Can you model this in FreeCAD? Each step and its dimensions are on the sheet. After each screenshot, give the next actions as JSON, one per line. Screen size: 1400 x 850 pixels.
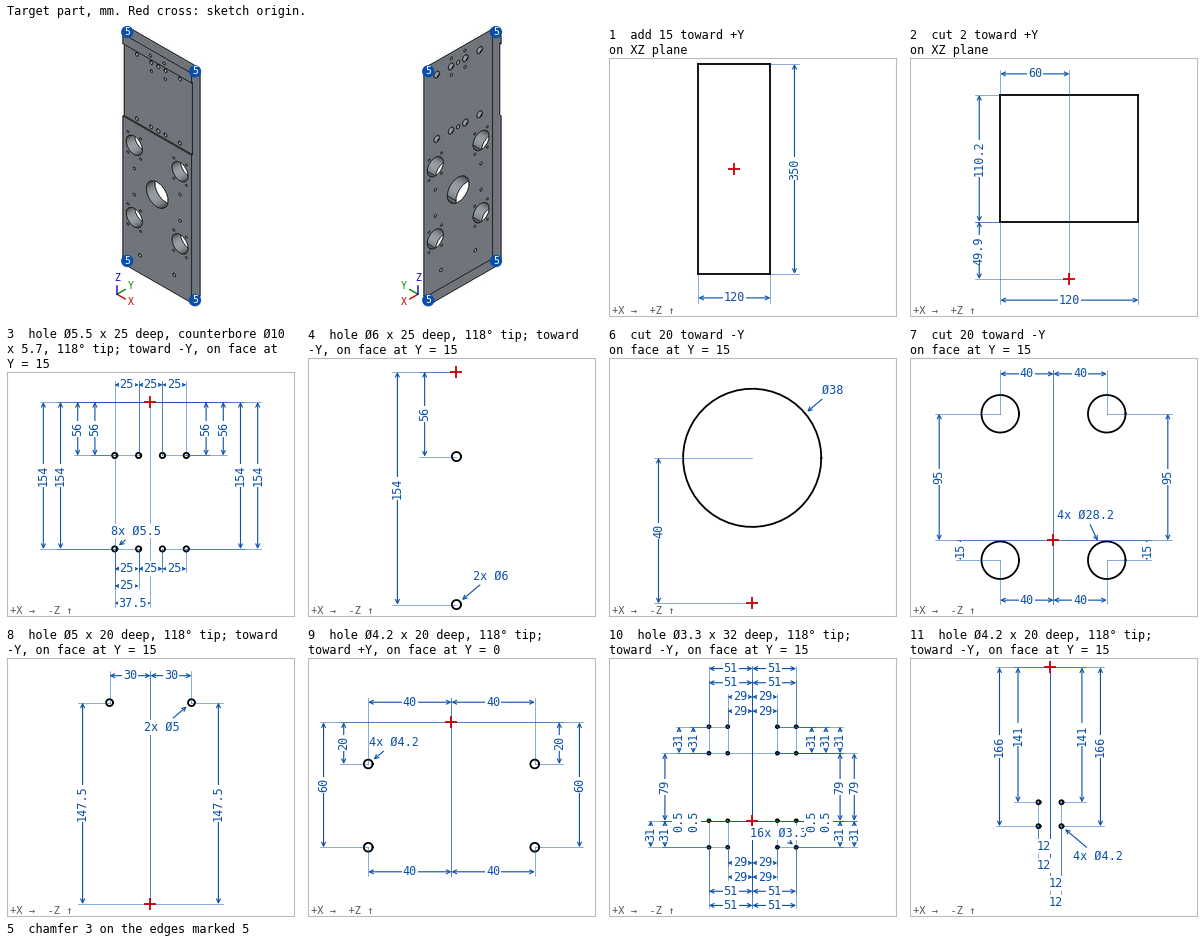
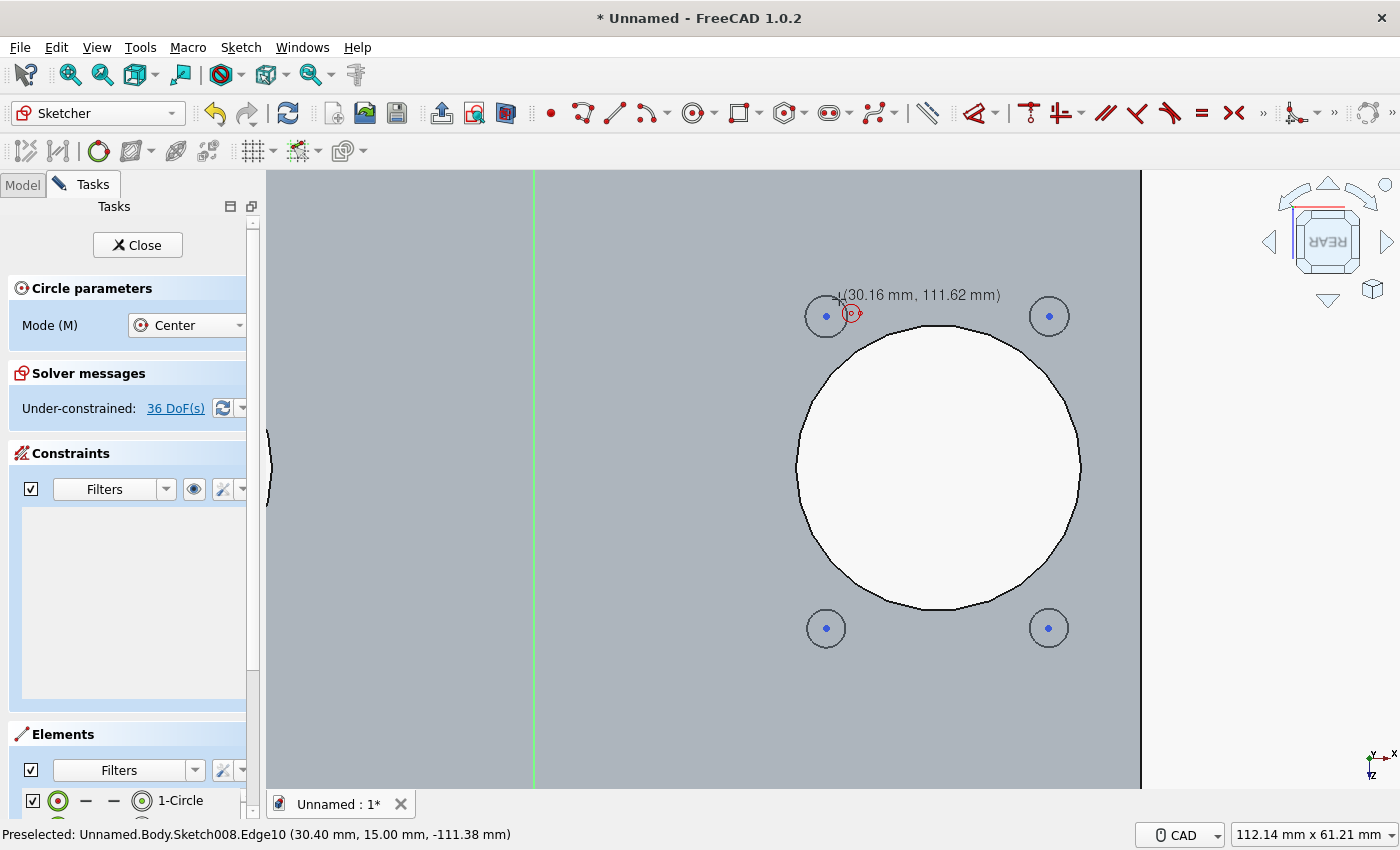
{"action": "scroll", "coordinate": [840, 301], "scroll_direction": "down", "scroll_amount": 7}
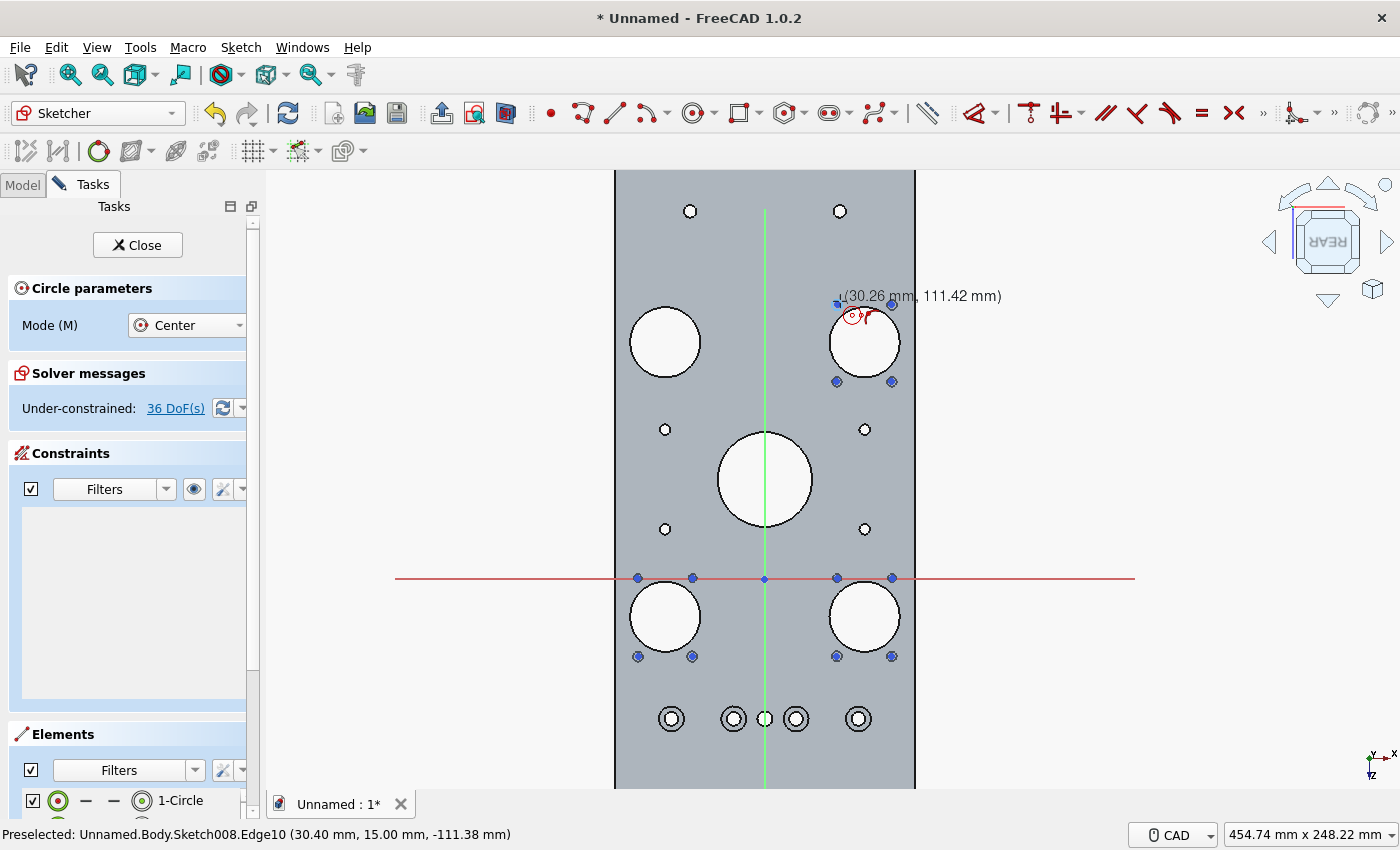
{"action": "scroll", "coordinate": [693, 381], "scroll_direction": "up", "scroll_amount": 9}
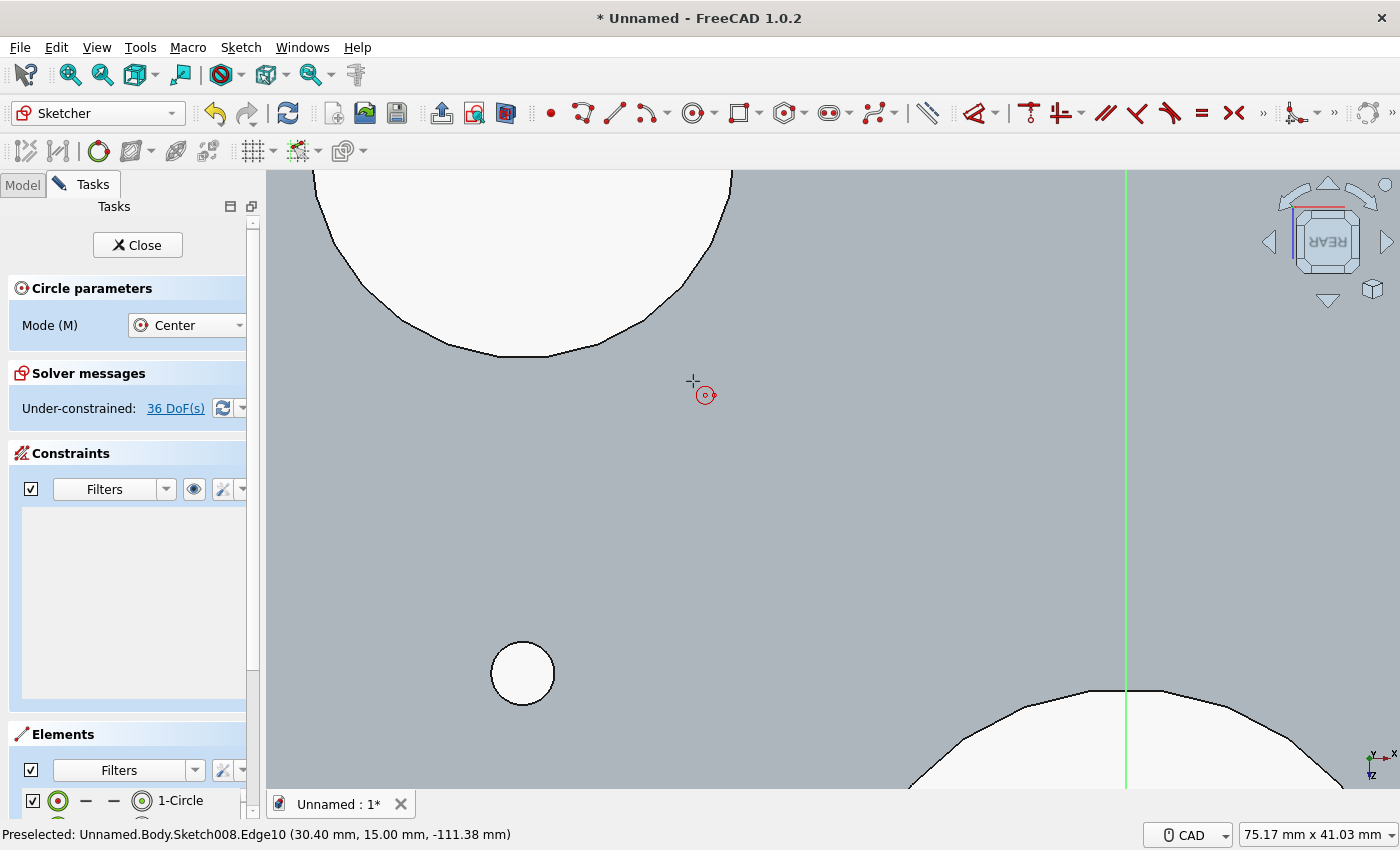
{"action": "scroll", "coordinate": [693, 381], "scroll_direction": "down", "scroll_amount": 9}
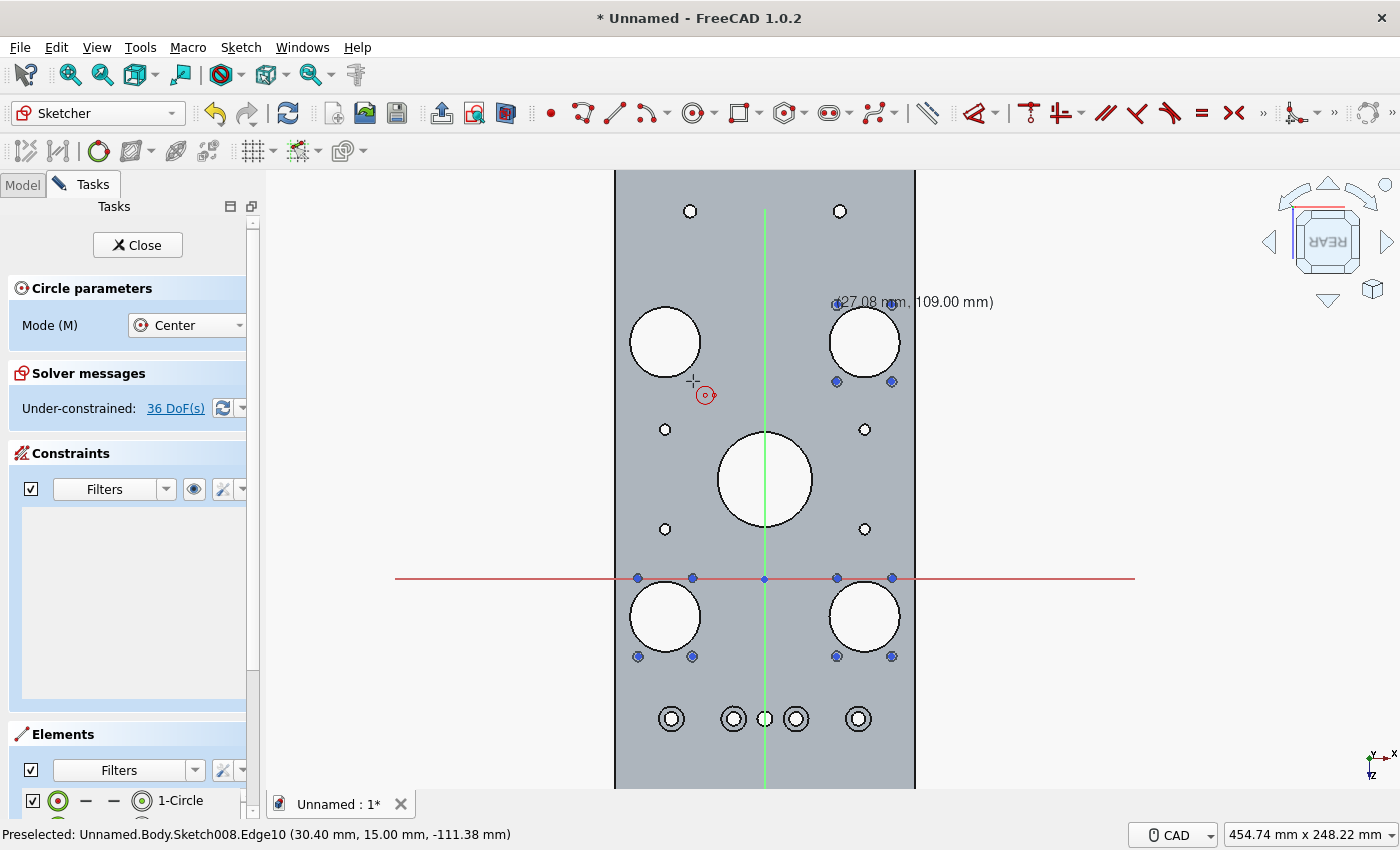
{"action": "left_click", "coordinate": [693, 381]}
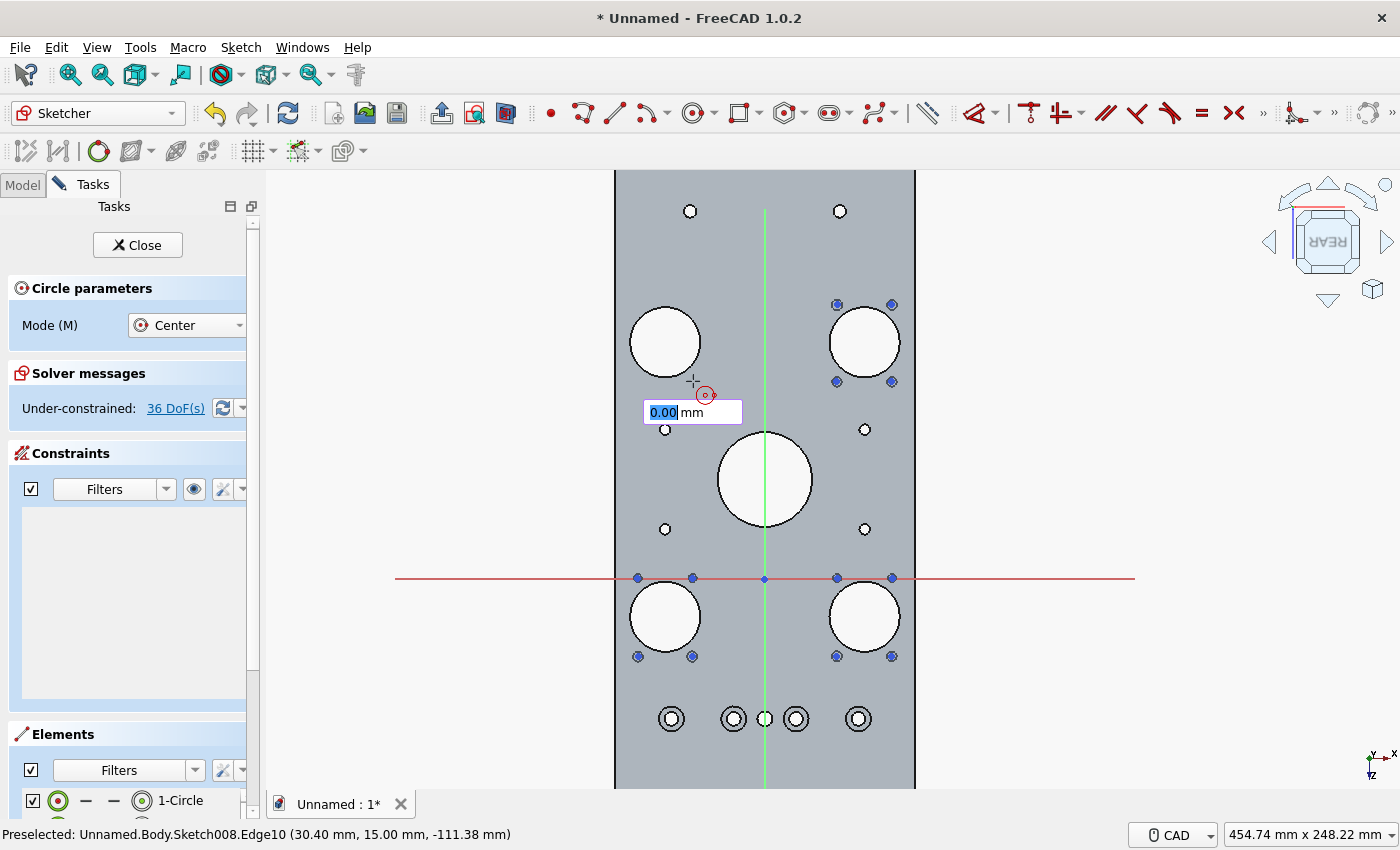
{"action": "scroll", "coordinate": [696, 378], "scroll_direction": "up", "scroll_amount": 7}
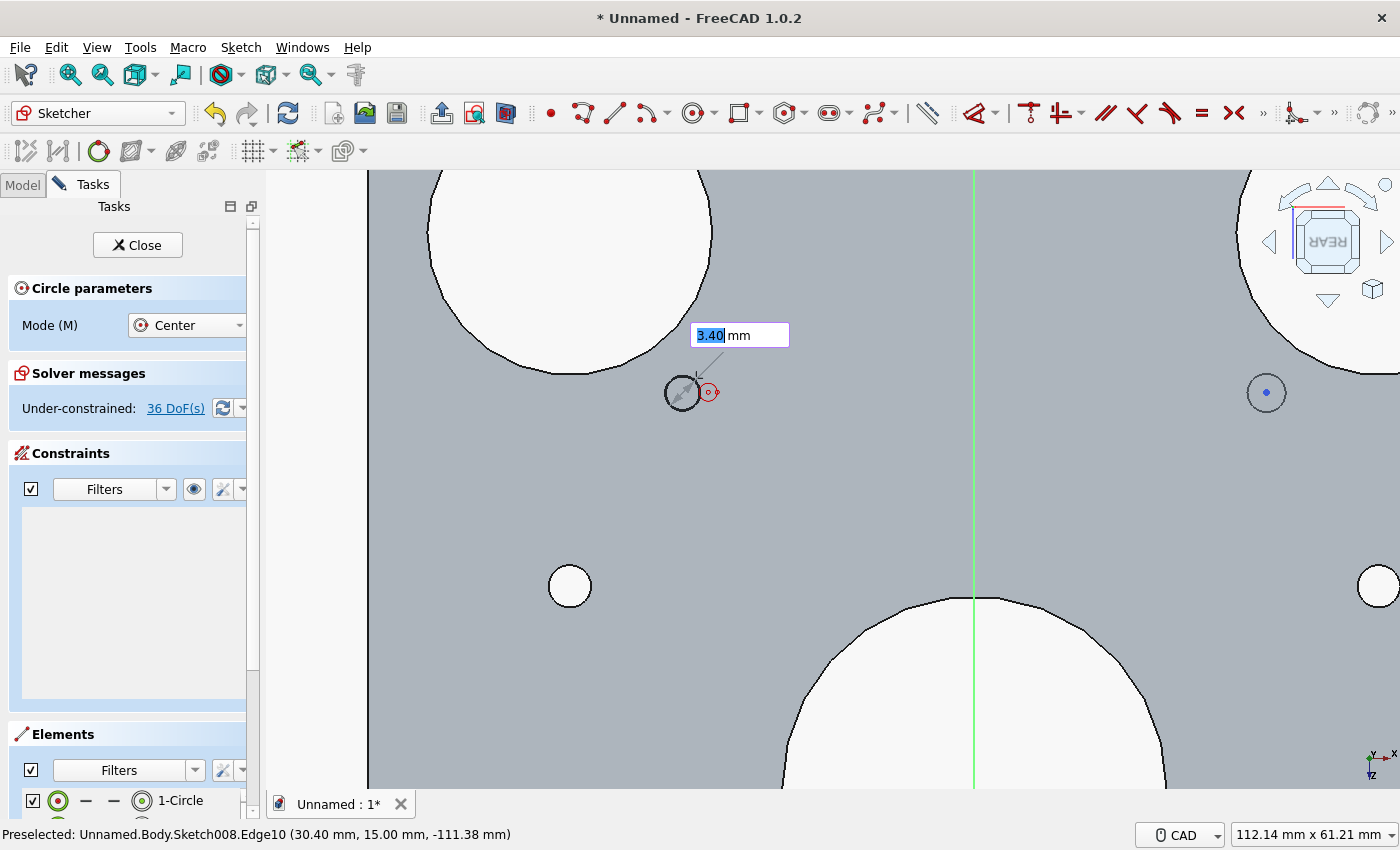
{"action": "left_click", "coordinate": [693, 377]}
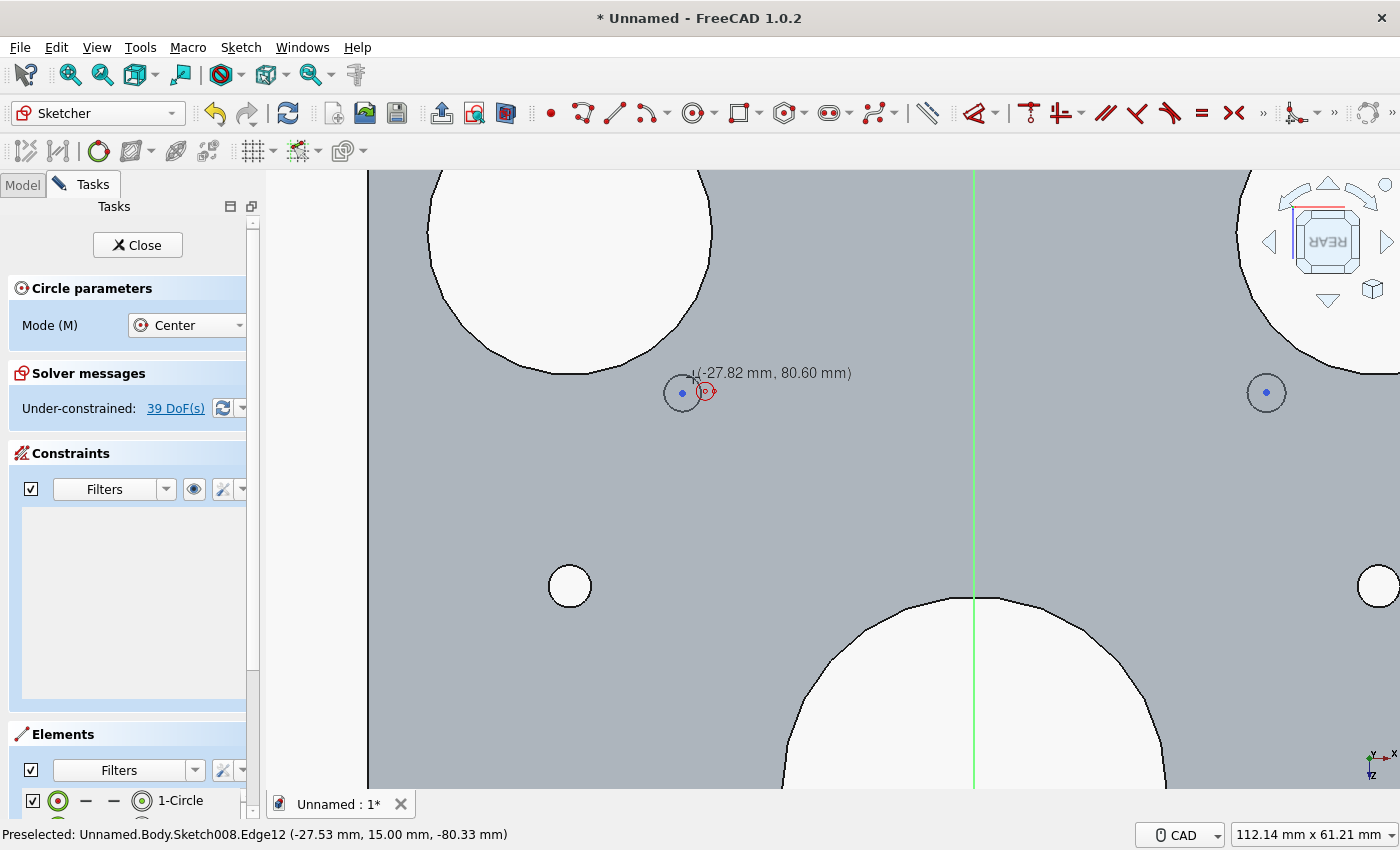
{"action": "scroll", "coordinate": [459, 389], "scroll_direction": "up", "scroll_amount": 2}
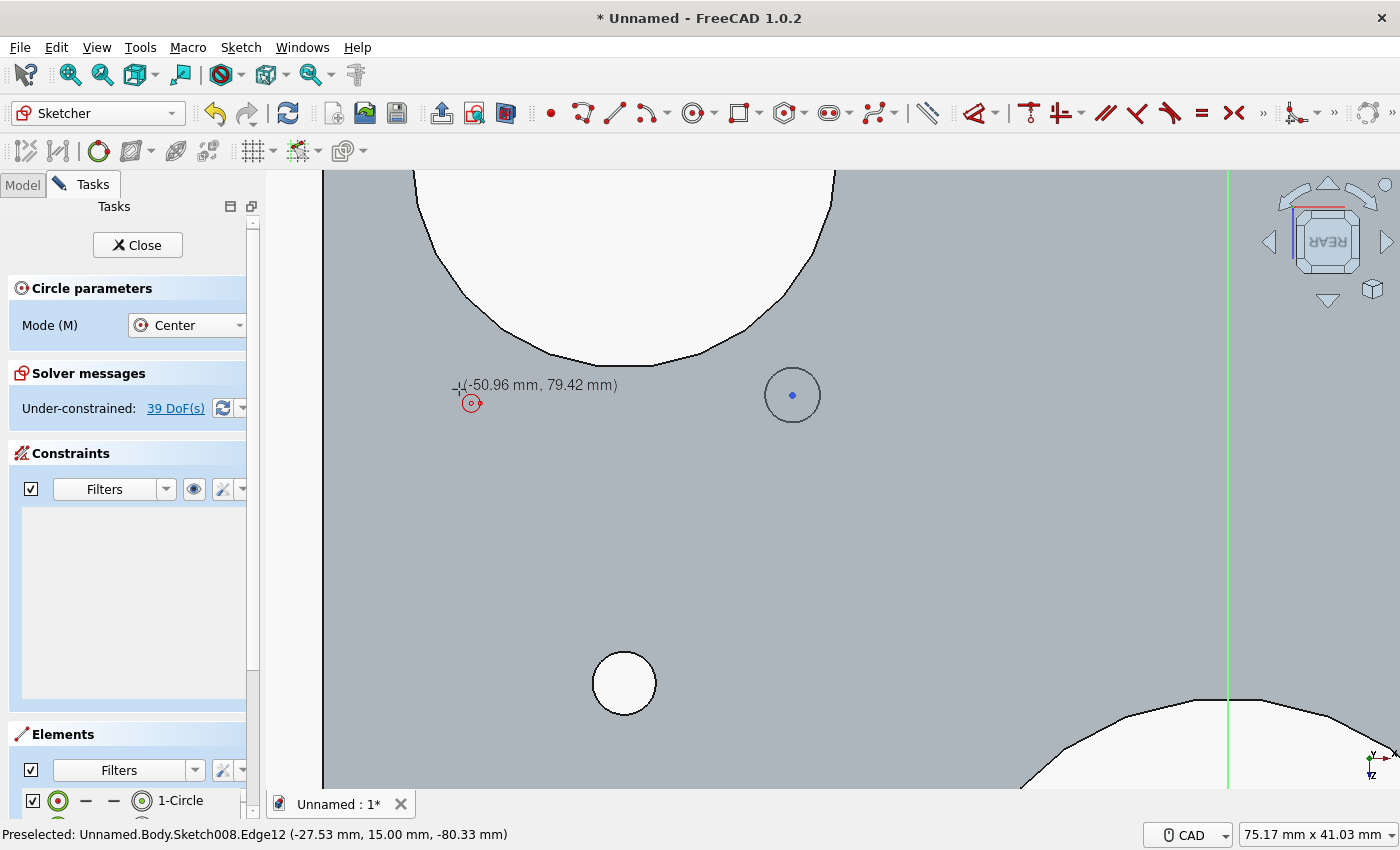
{"action": "scroll", "coordinate": [673, 379], "scroll_direction": "down", "scroll_amount": 9}